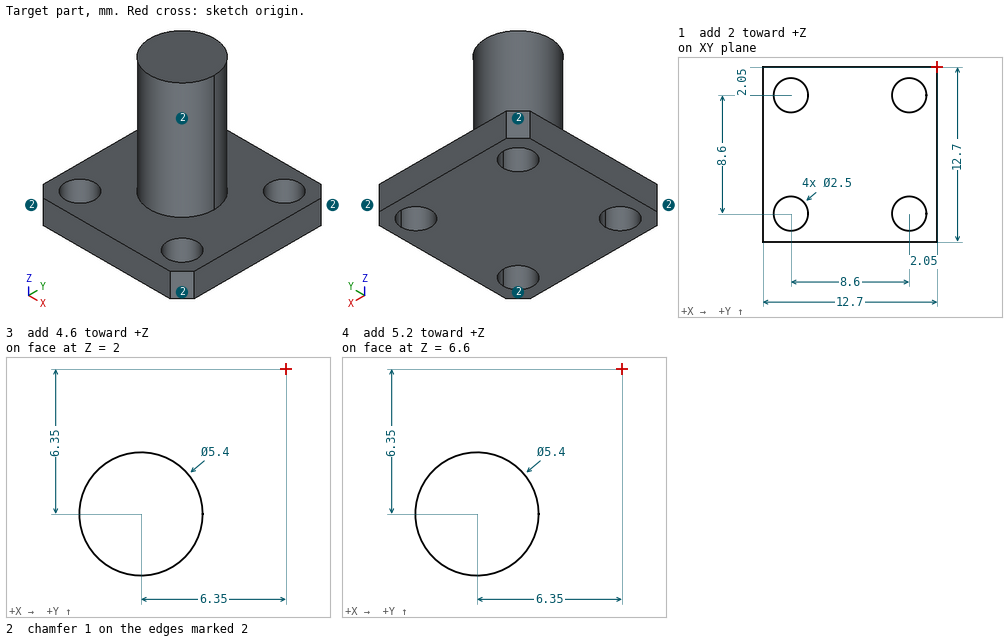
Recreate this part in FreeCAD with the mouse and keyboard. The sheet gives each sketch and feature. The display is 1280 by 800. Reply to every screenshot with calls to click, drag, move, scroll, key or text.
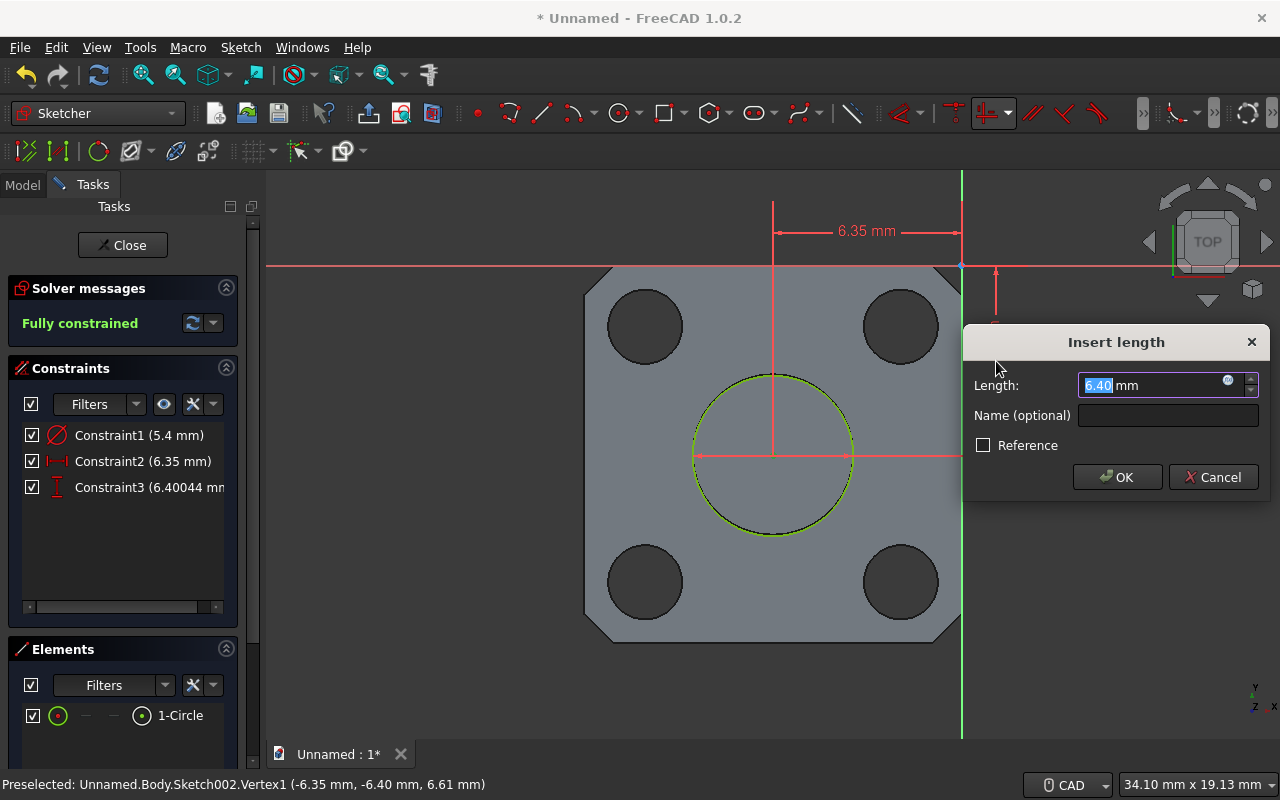
text(6.35)
key(Return)
key(Escape)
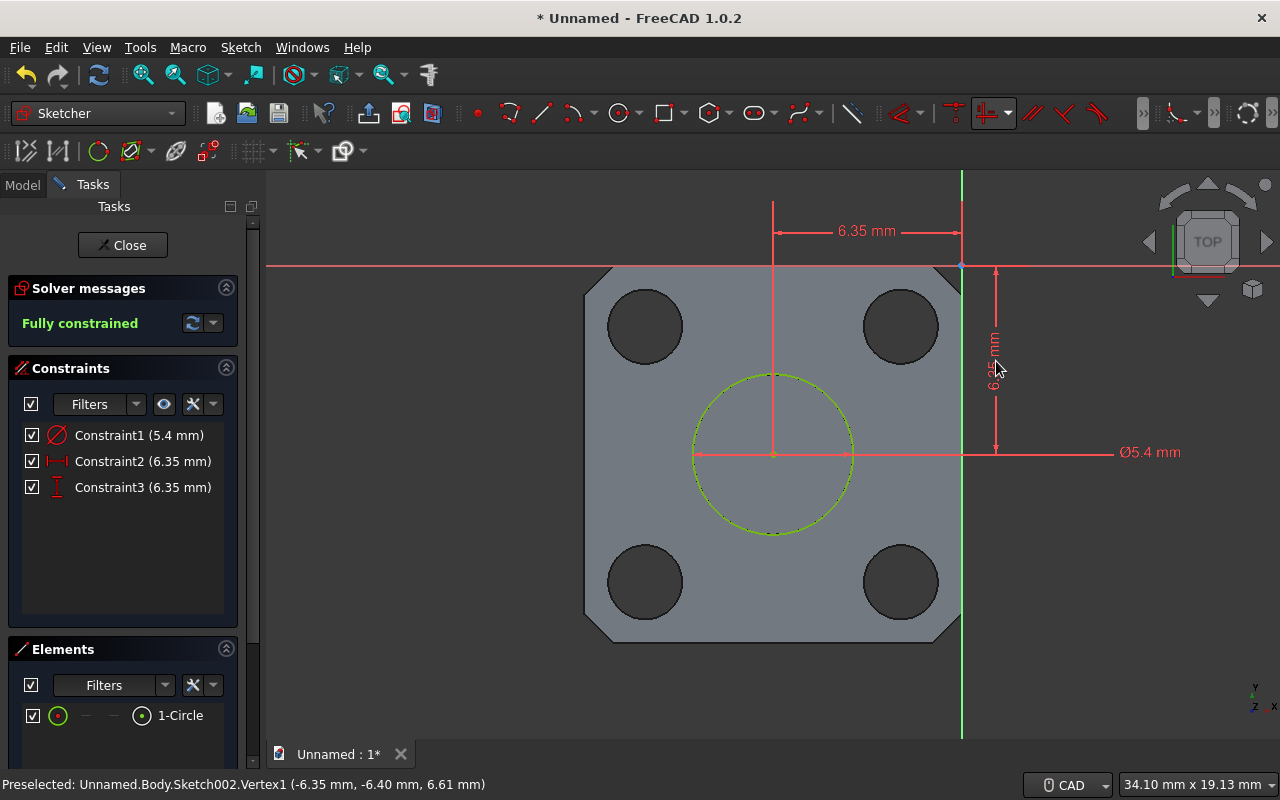
click(123, 245)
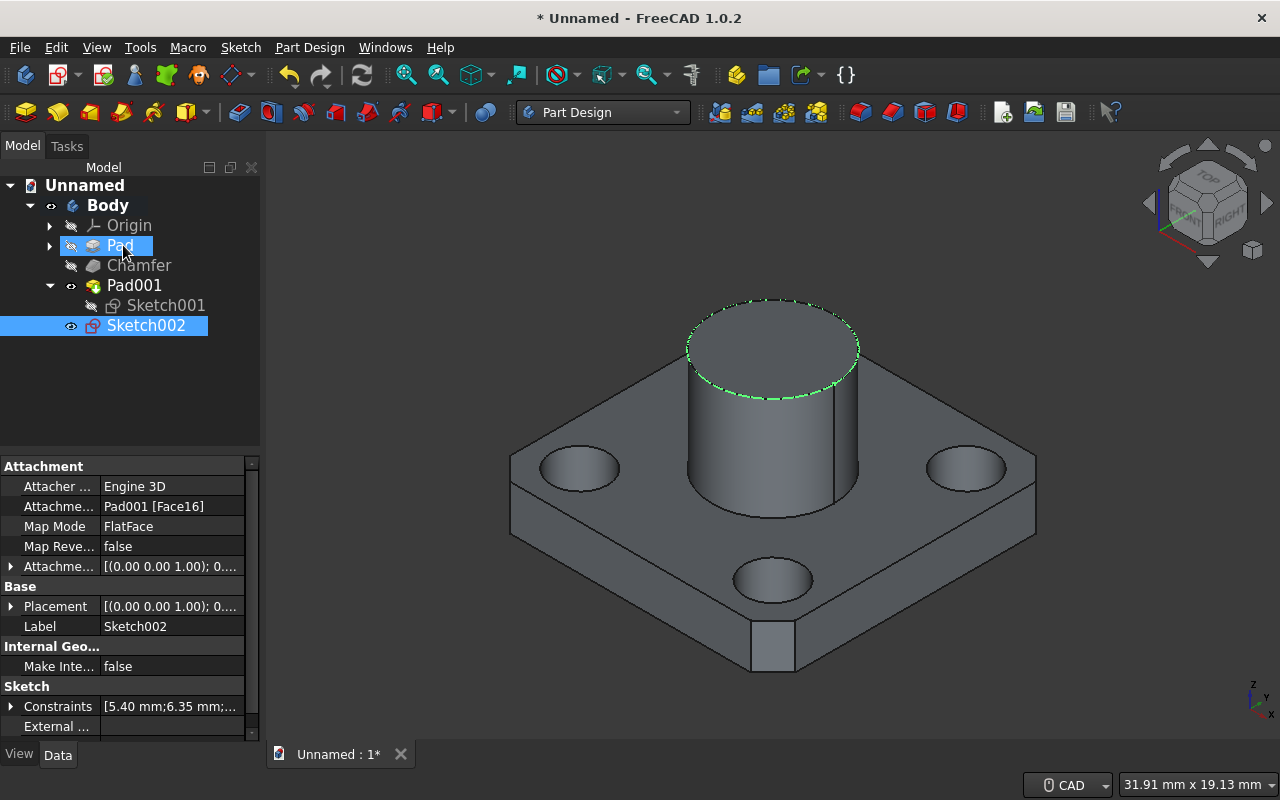
click(26, 112)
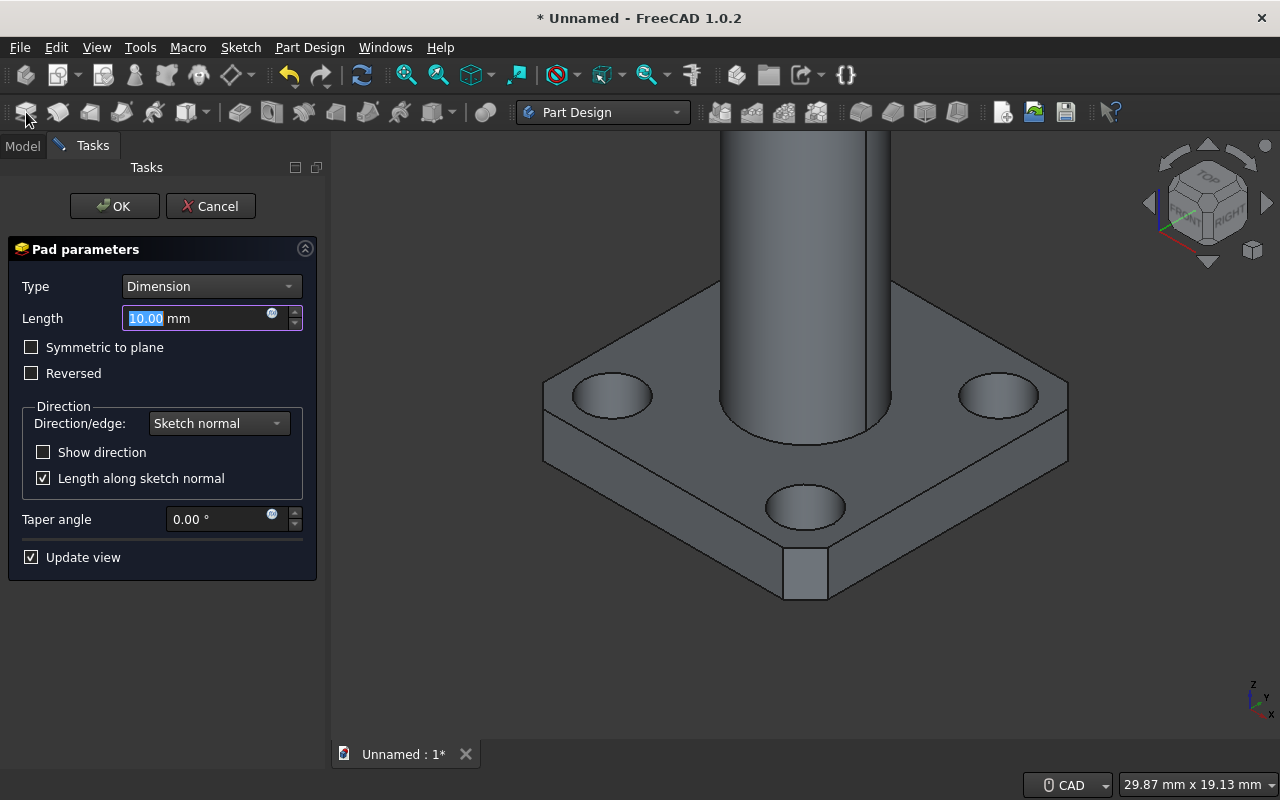
text(5.2)
key(Tab)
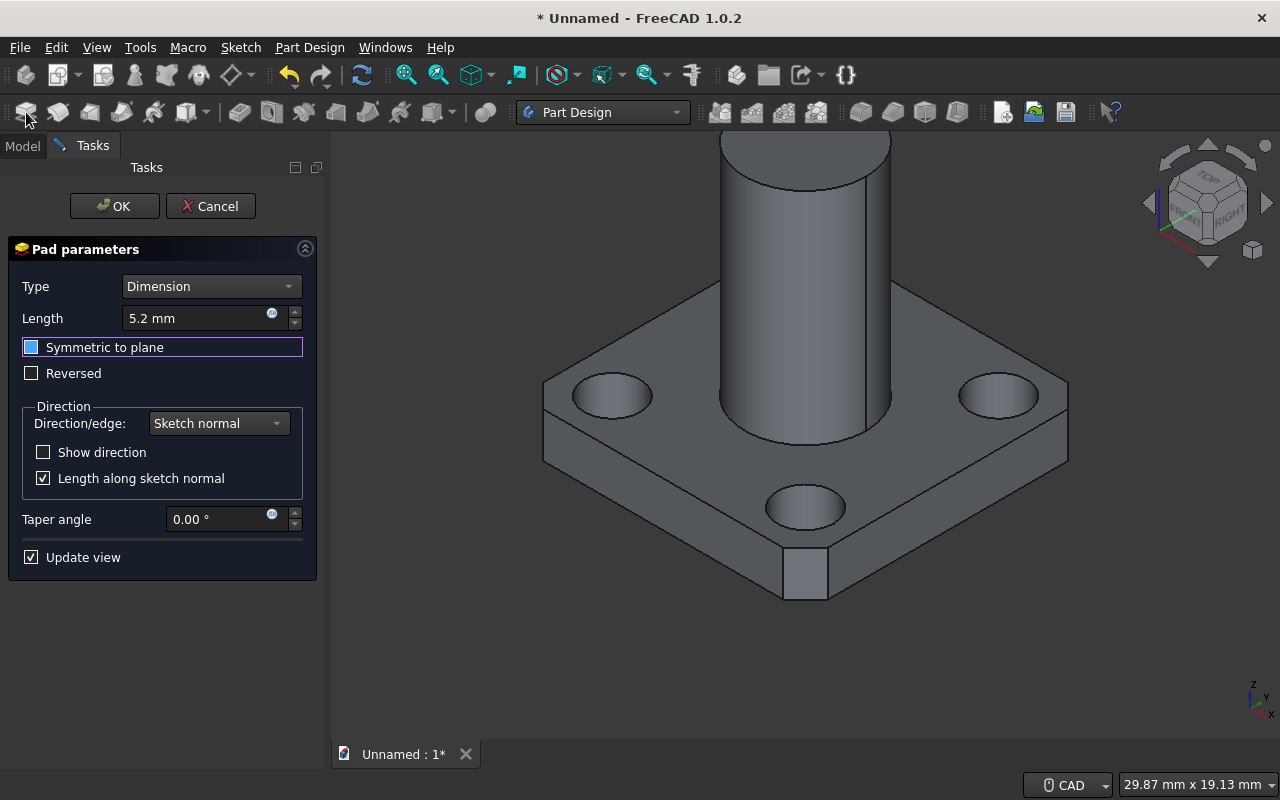
click(115, 206)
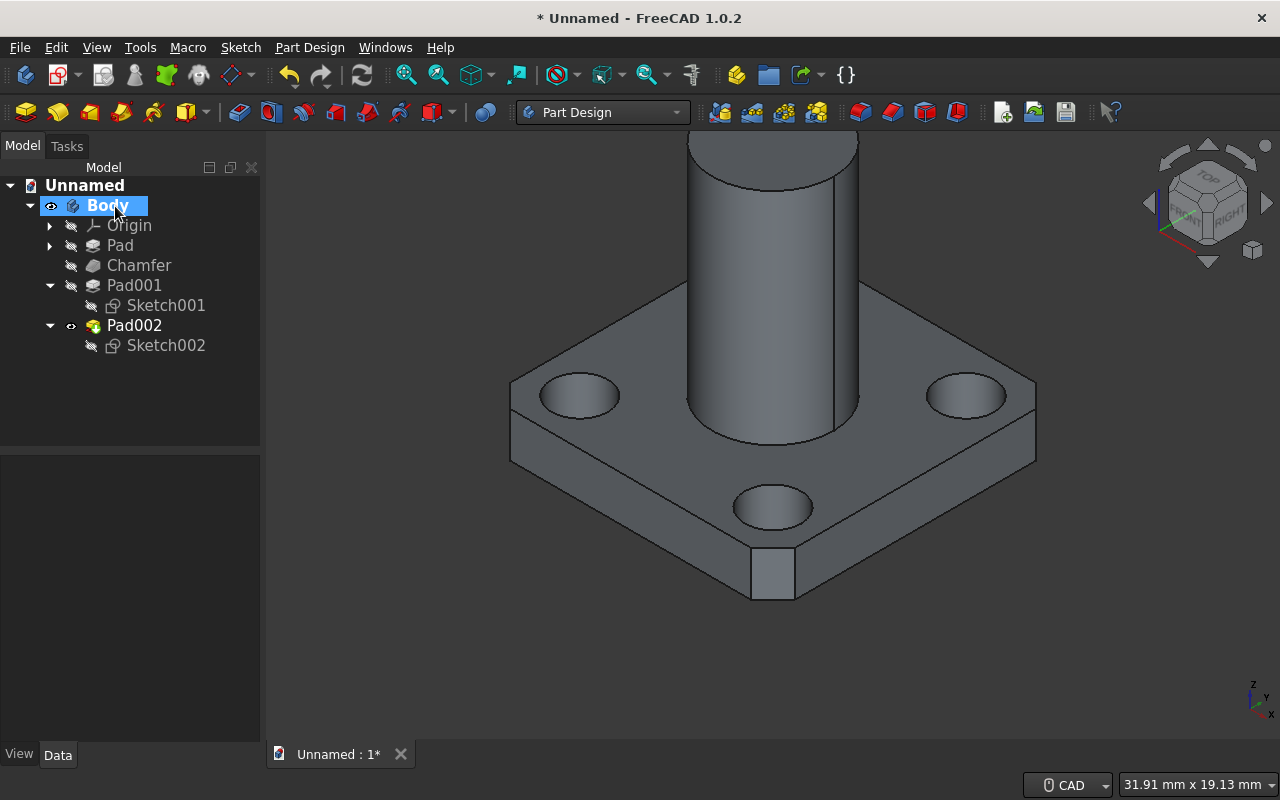
click(408, 76)